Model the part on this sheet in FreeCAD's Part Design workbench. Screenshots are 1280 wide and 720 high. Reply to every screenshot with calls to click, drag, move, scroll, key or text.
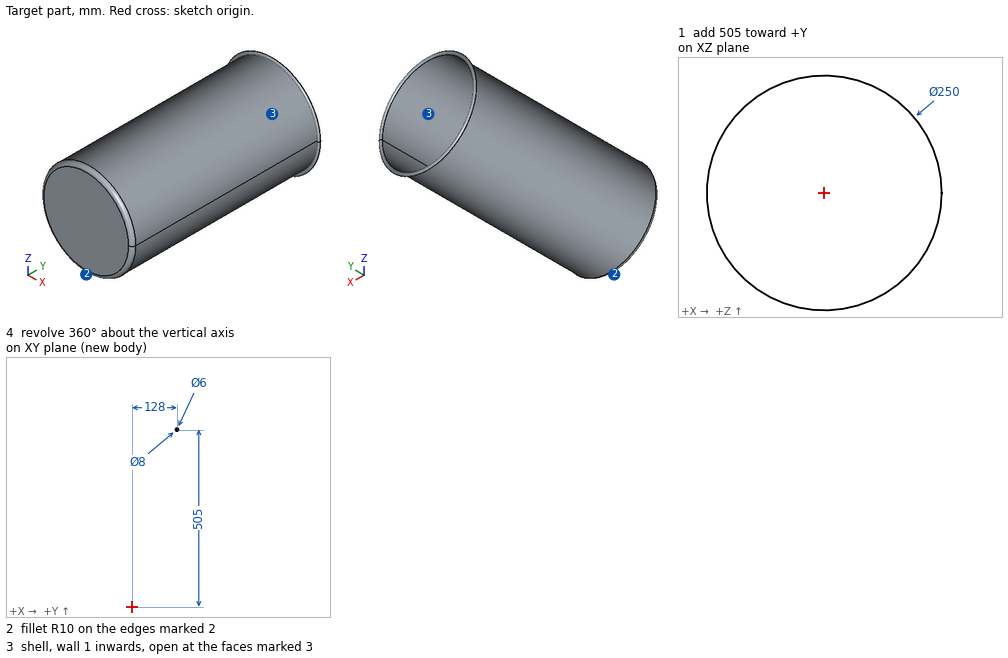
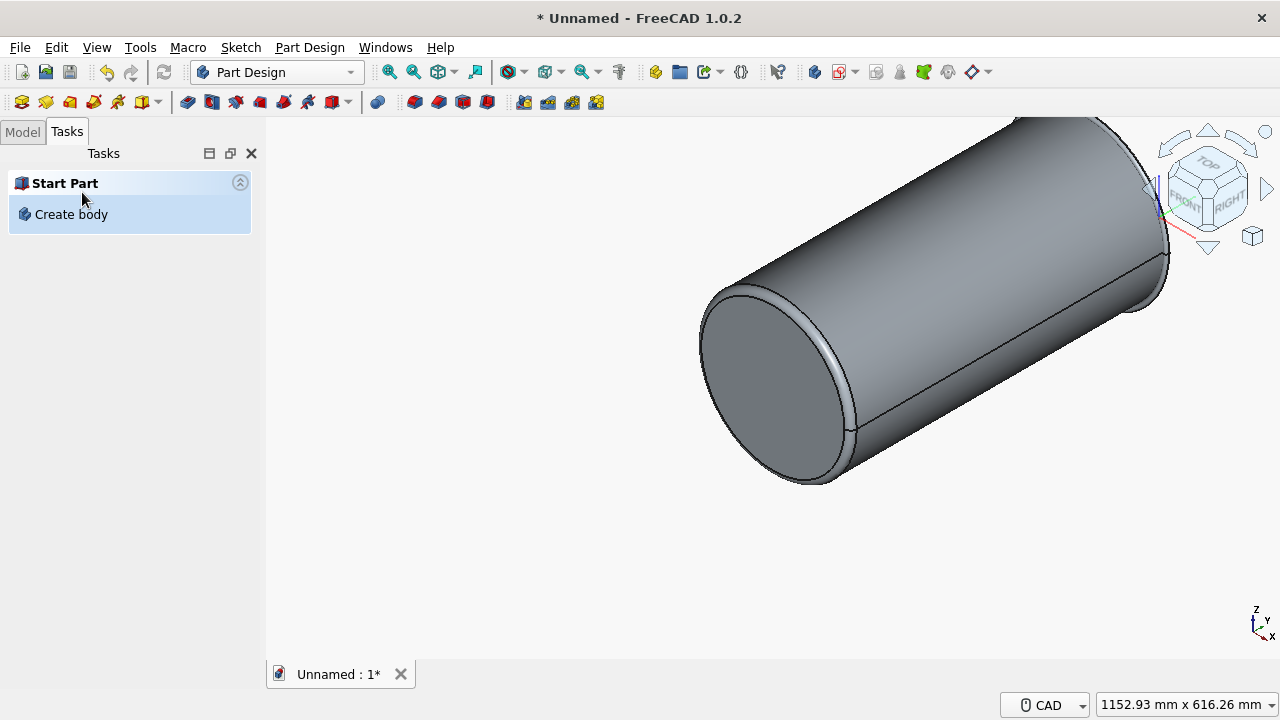
click(390, 72)